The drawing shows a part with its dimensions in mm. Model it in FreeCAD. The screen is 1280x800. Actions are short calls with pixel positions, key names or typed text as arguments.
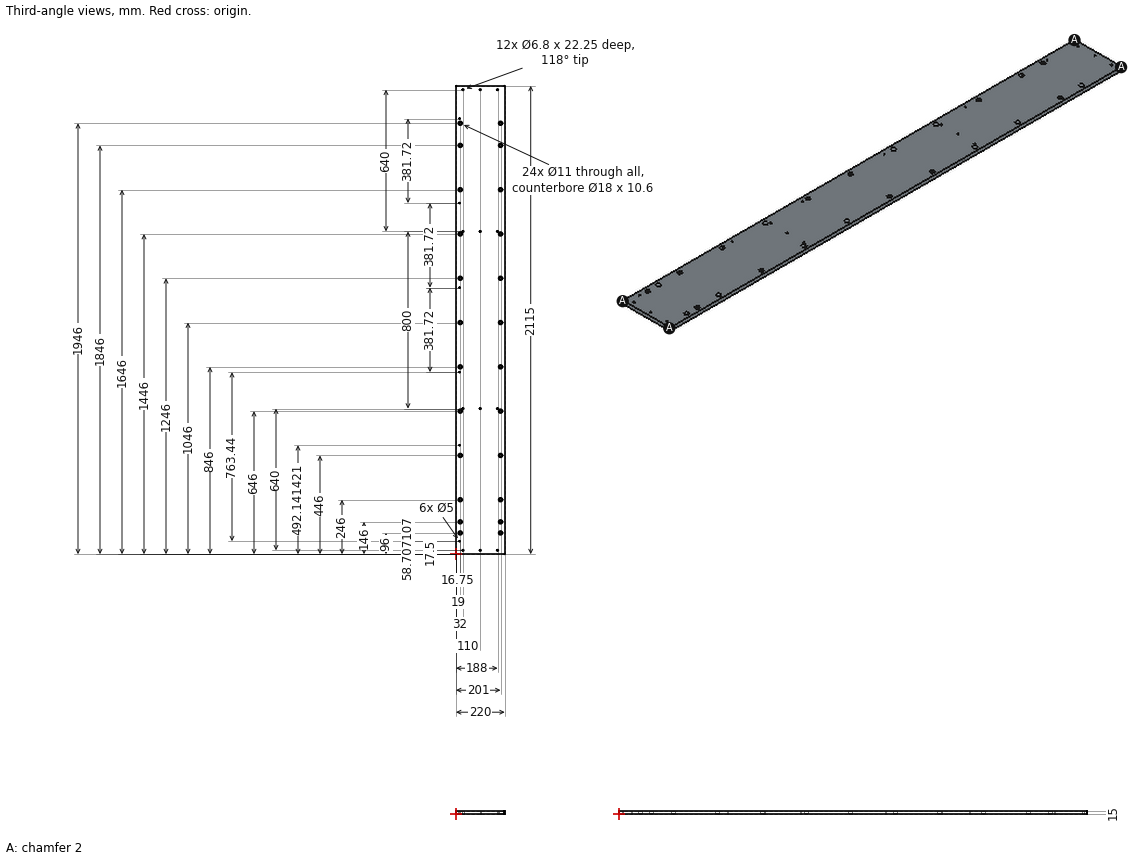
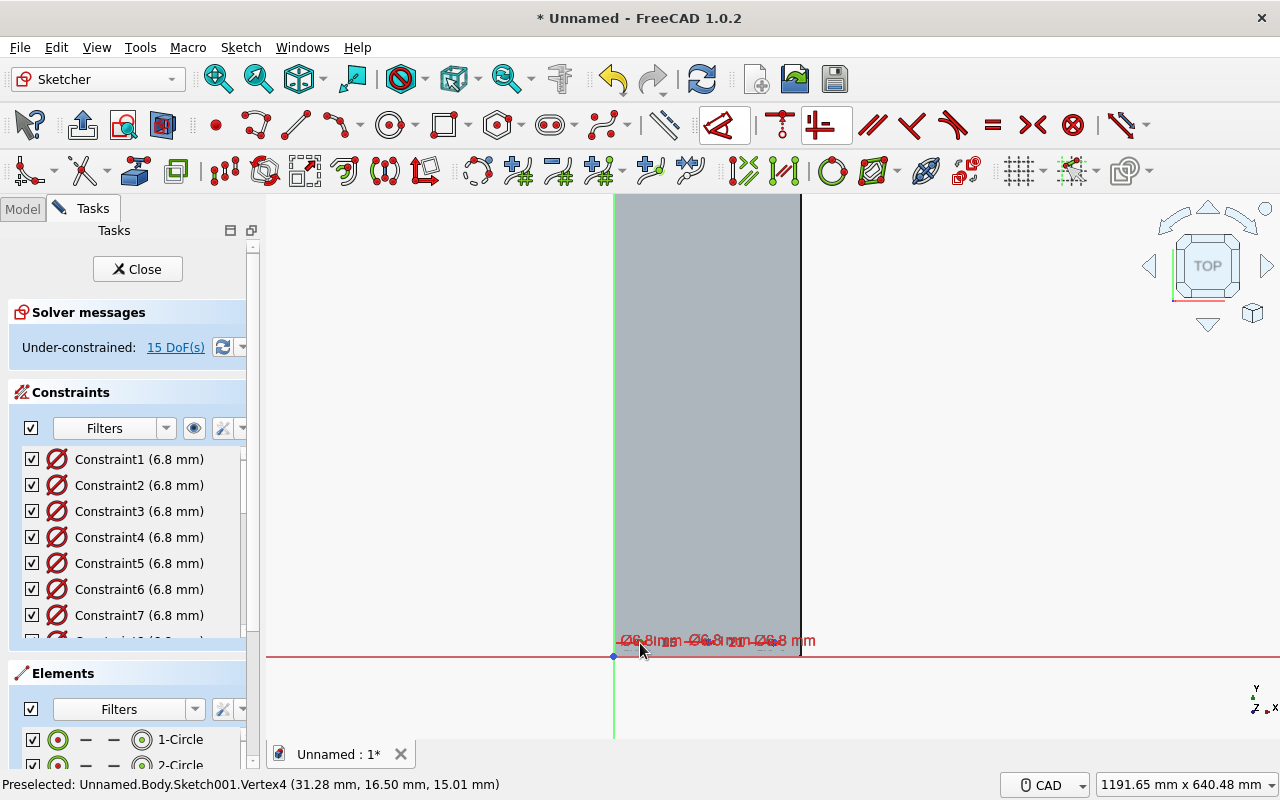
scroll(707, 645, down, 8)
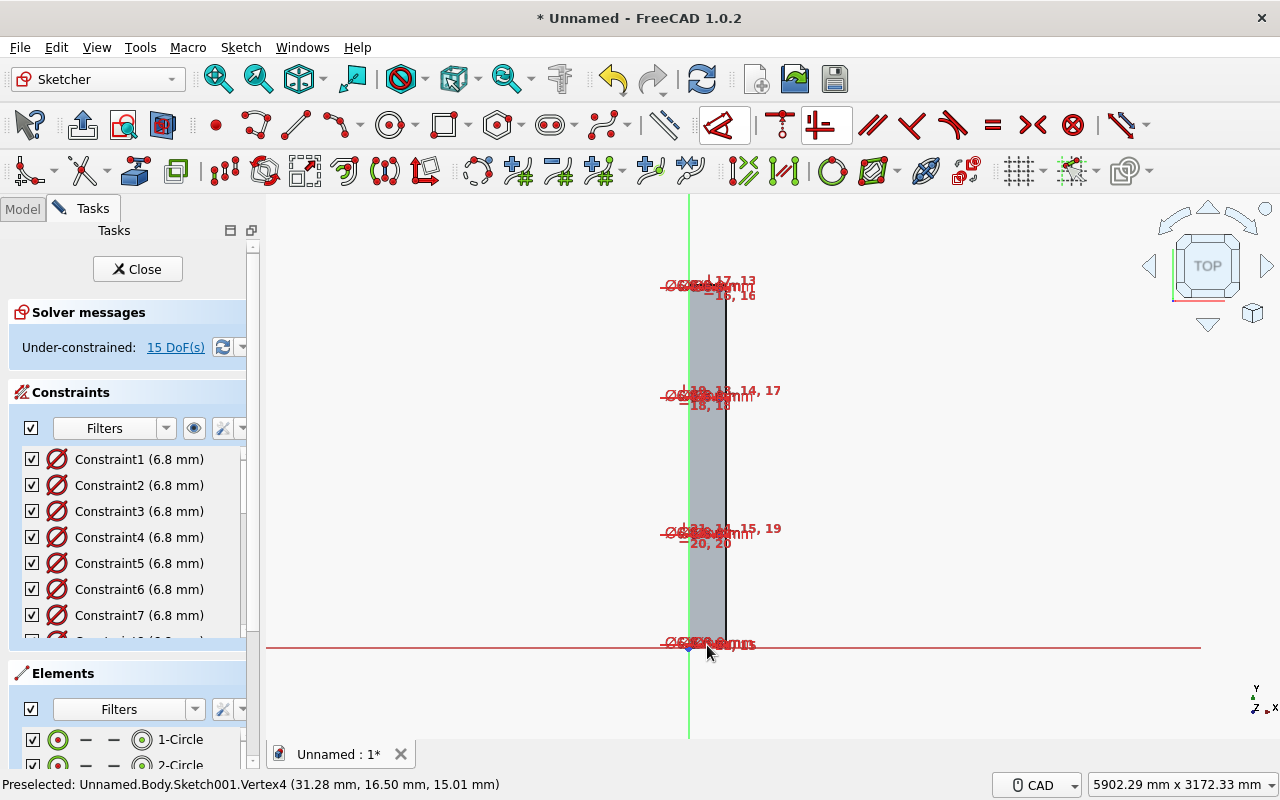
scroll(708, 645, up, 4)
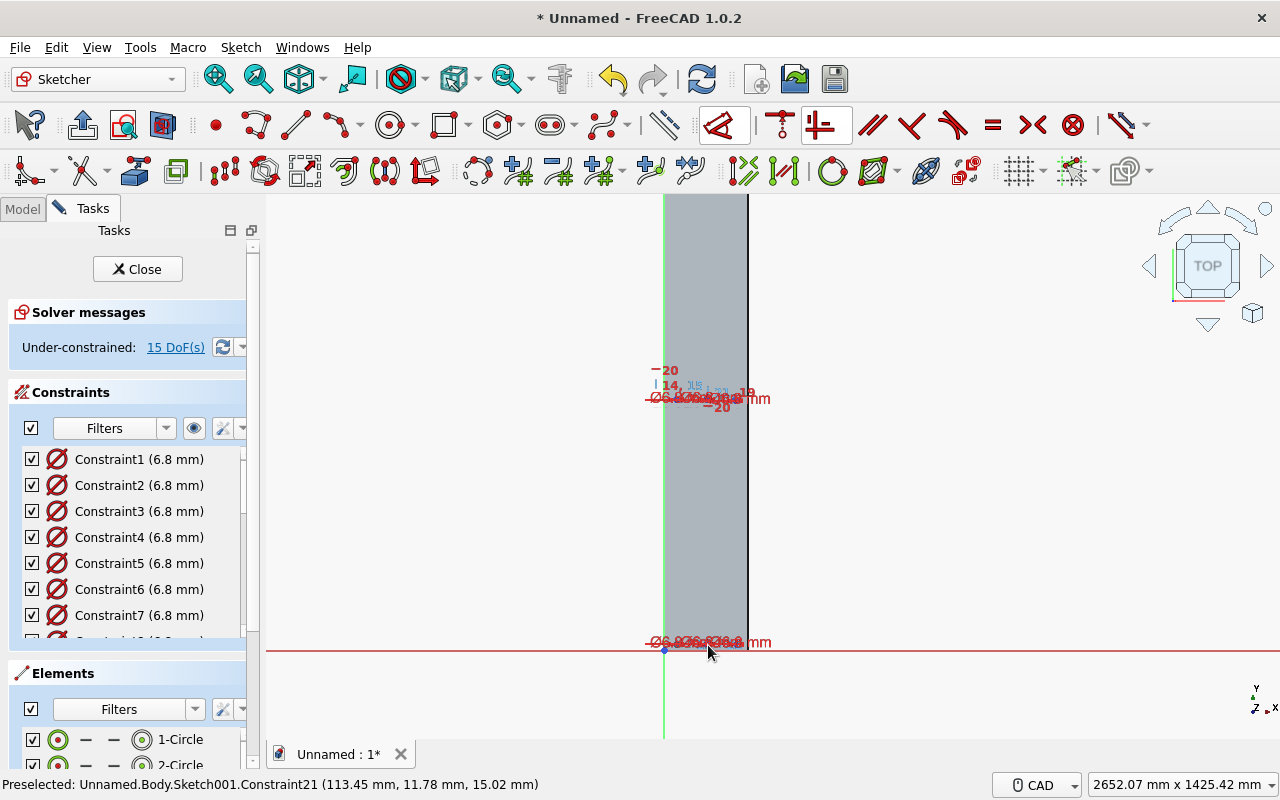
scroll(707, 644, up, 4)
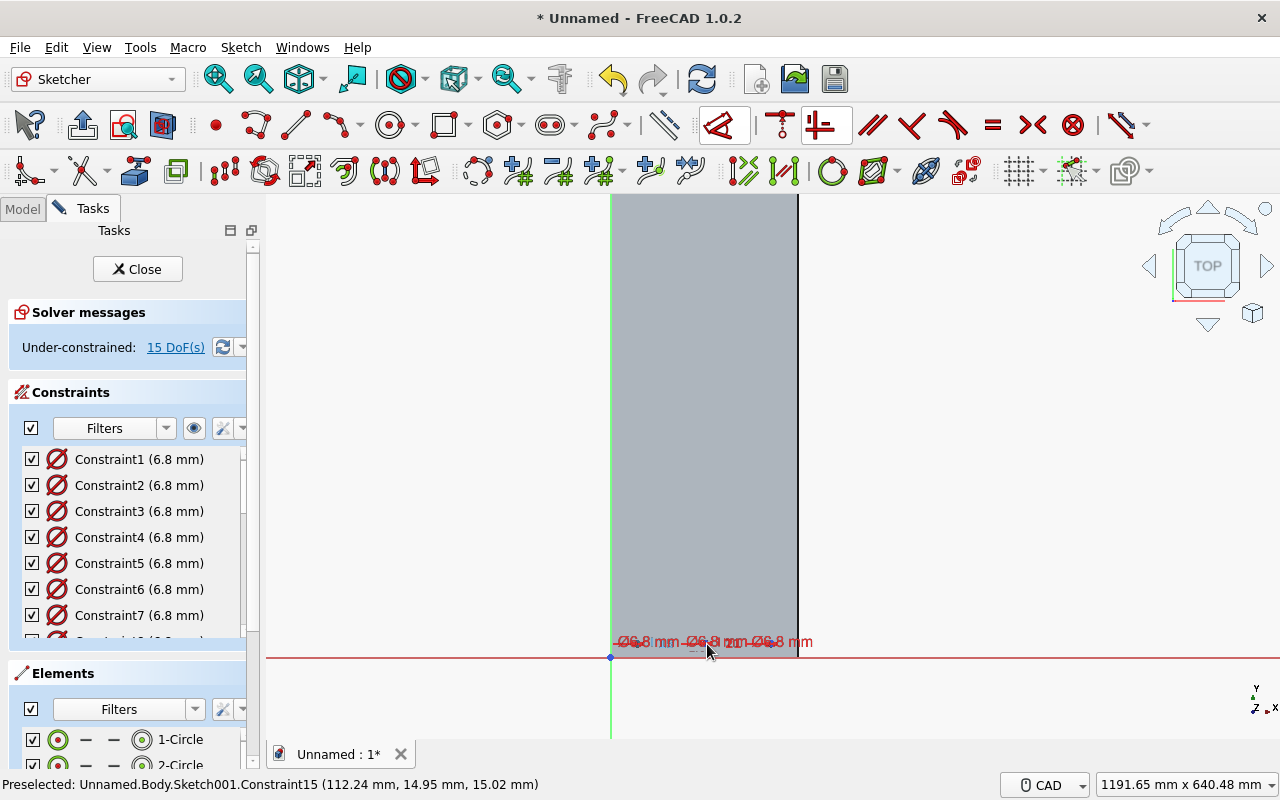
click(706, 644)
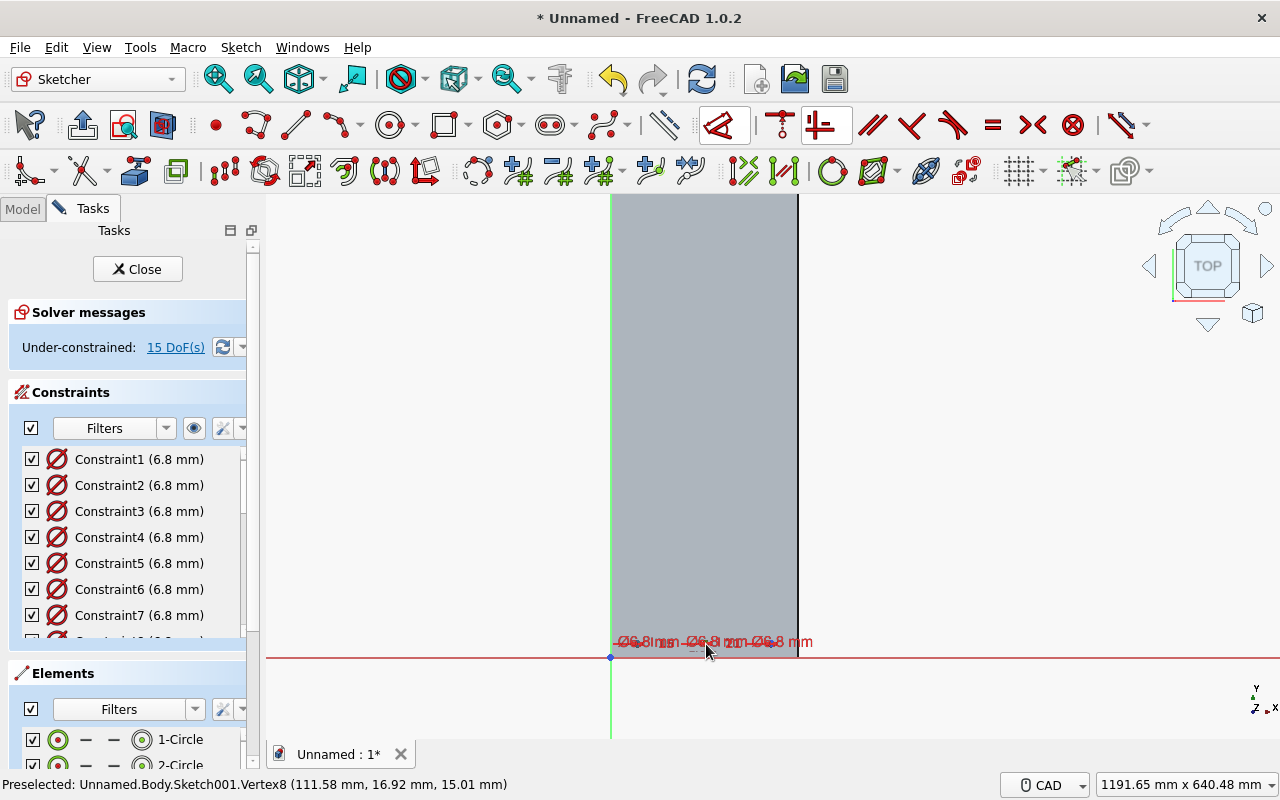
key(h)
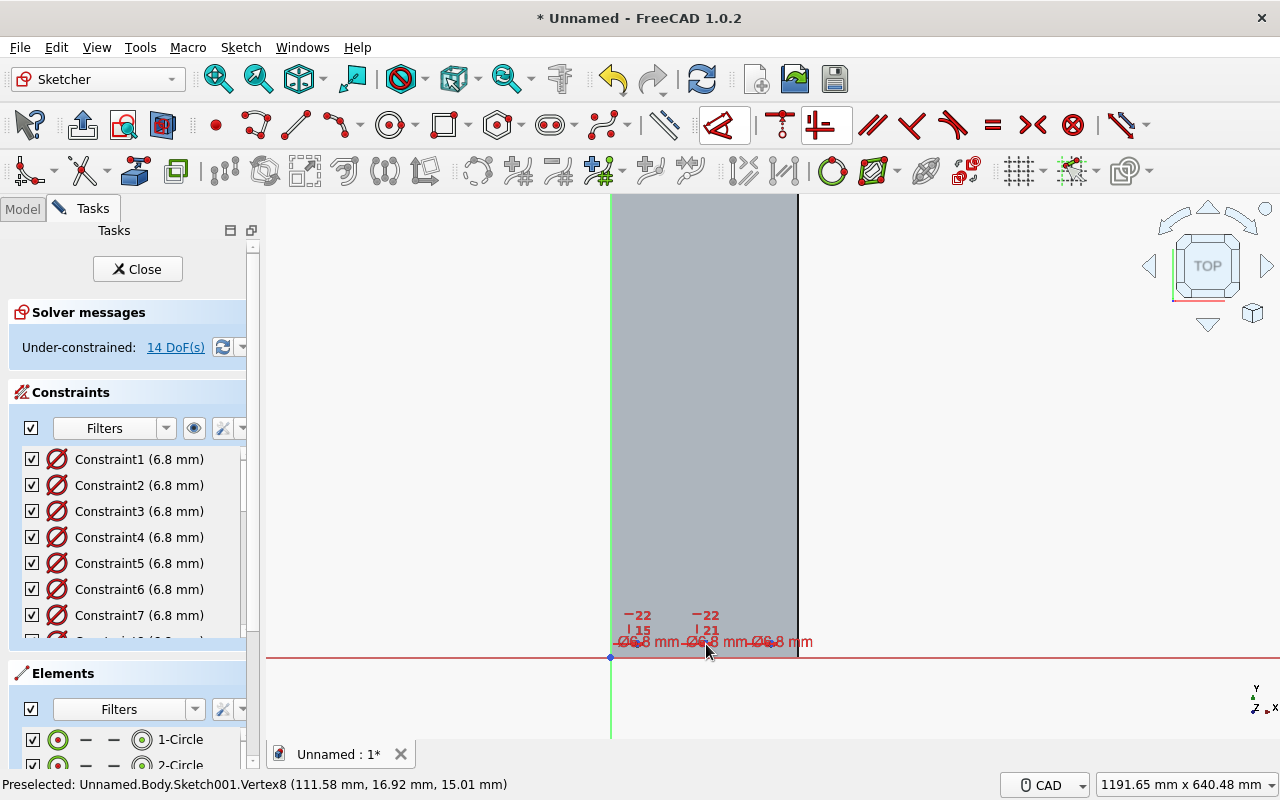
scroll(708, 644, down, 8)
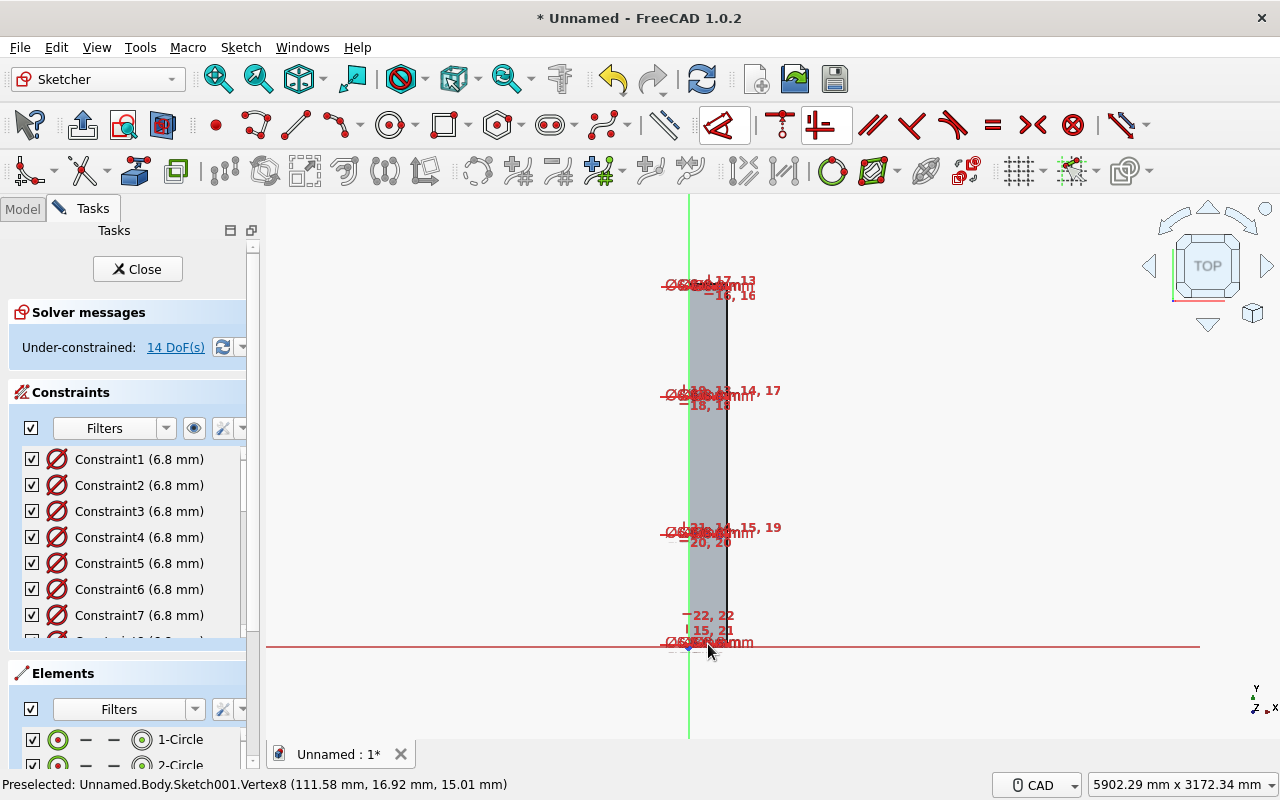
click(708, 287)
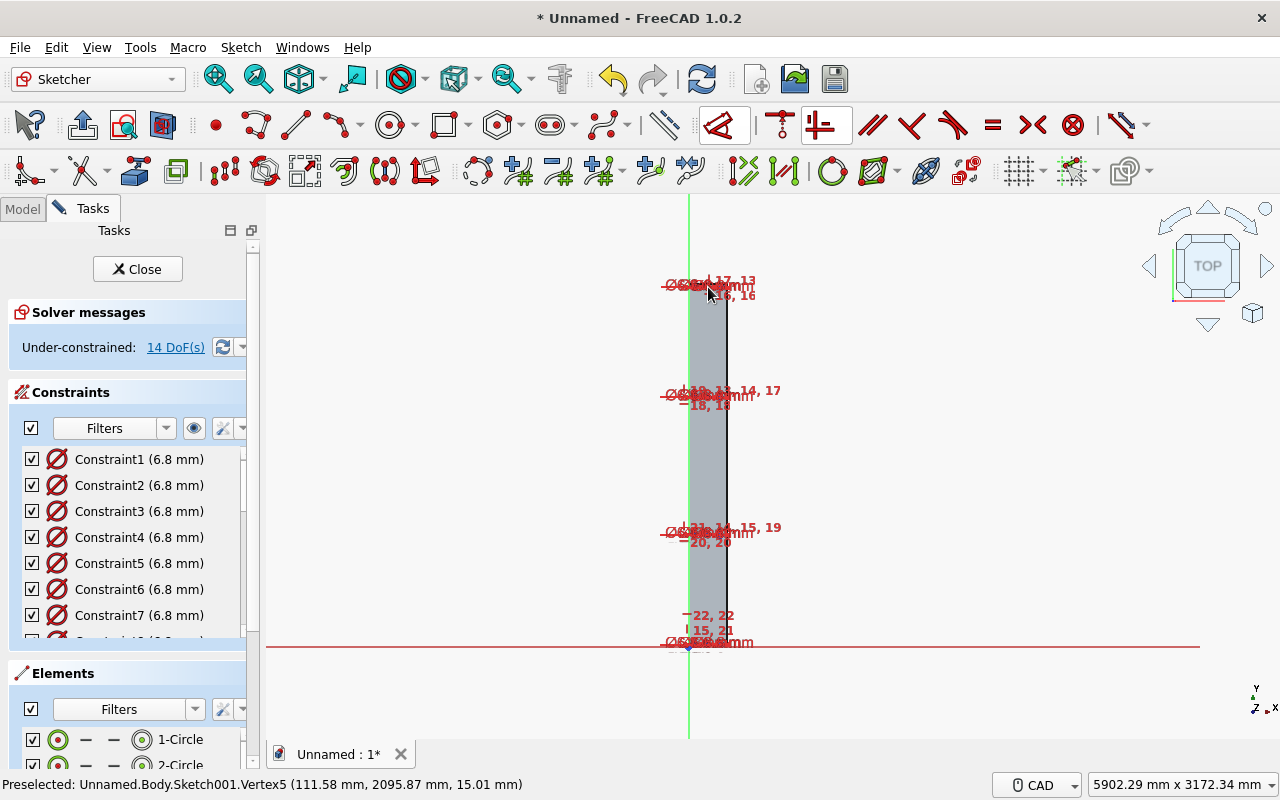
click(721, 288)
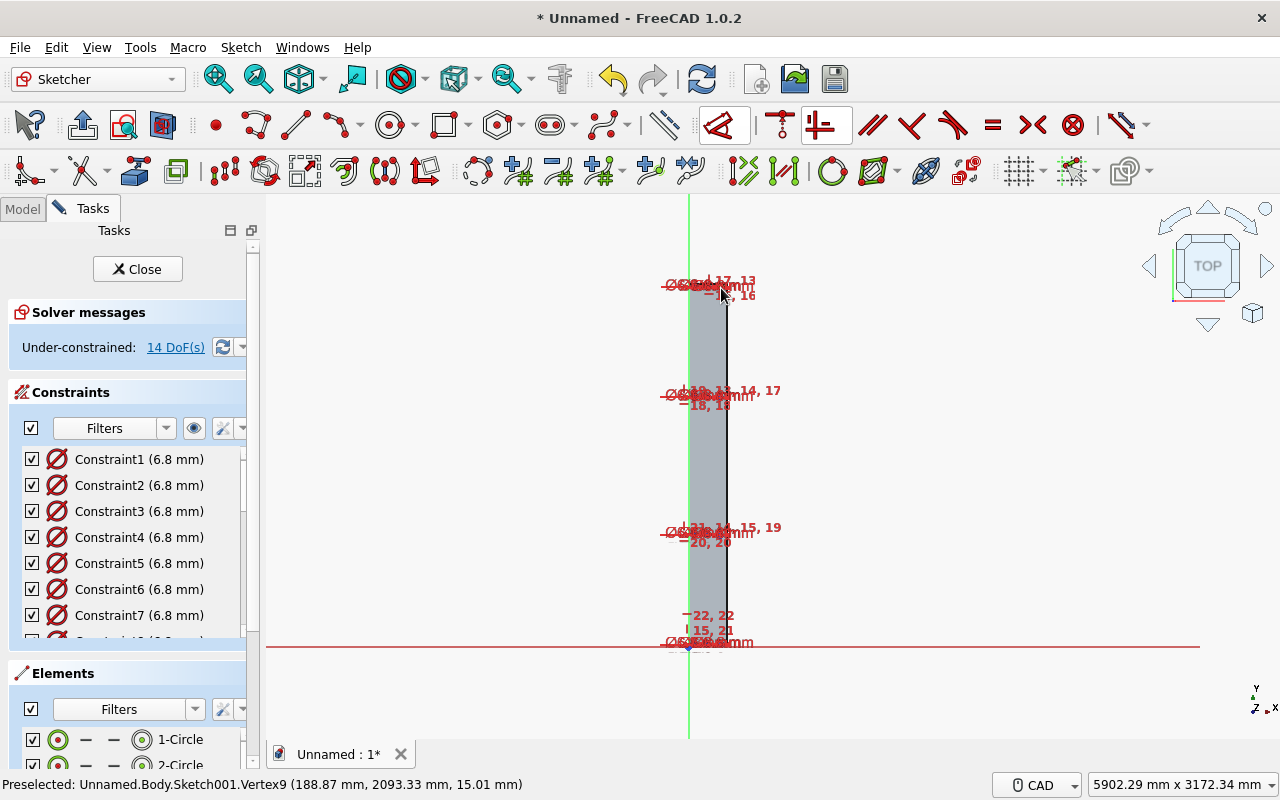
click(846, 126)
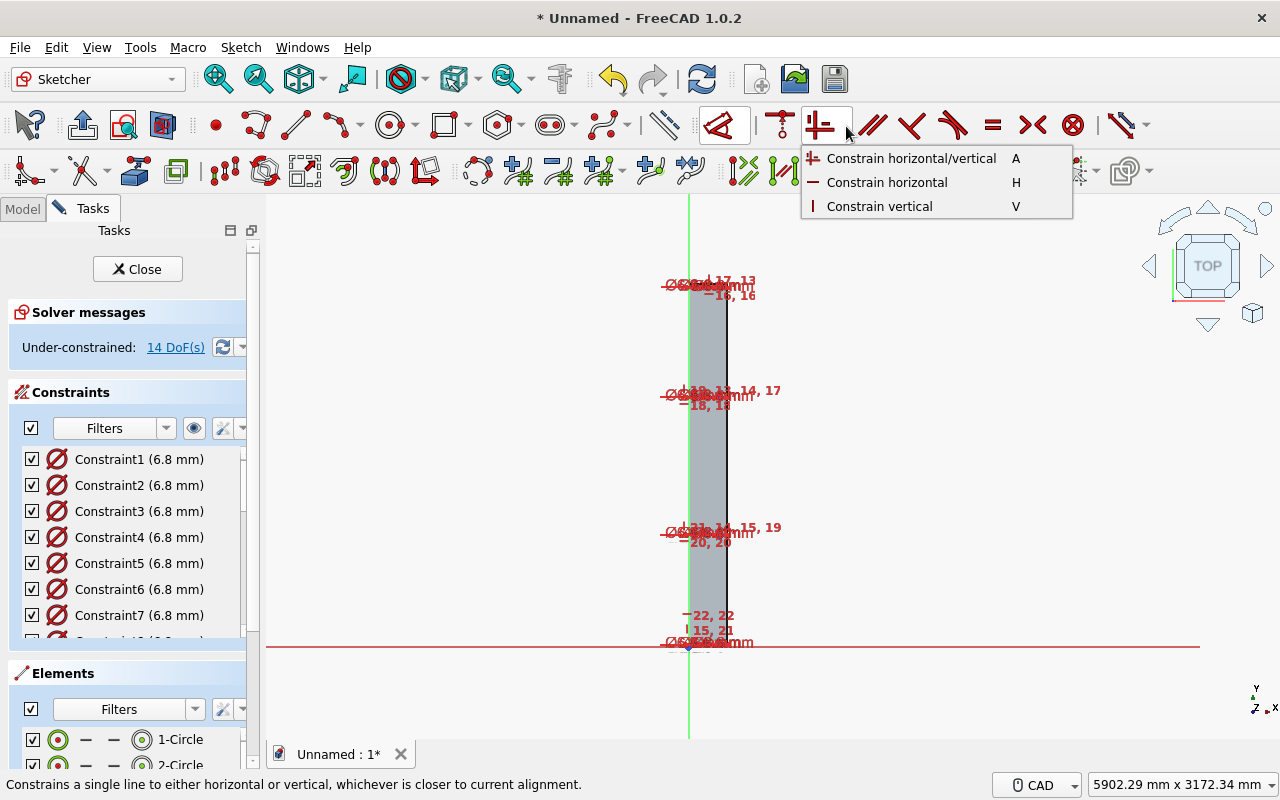
click(937, 182)